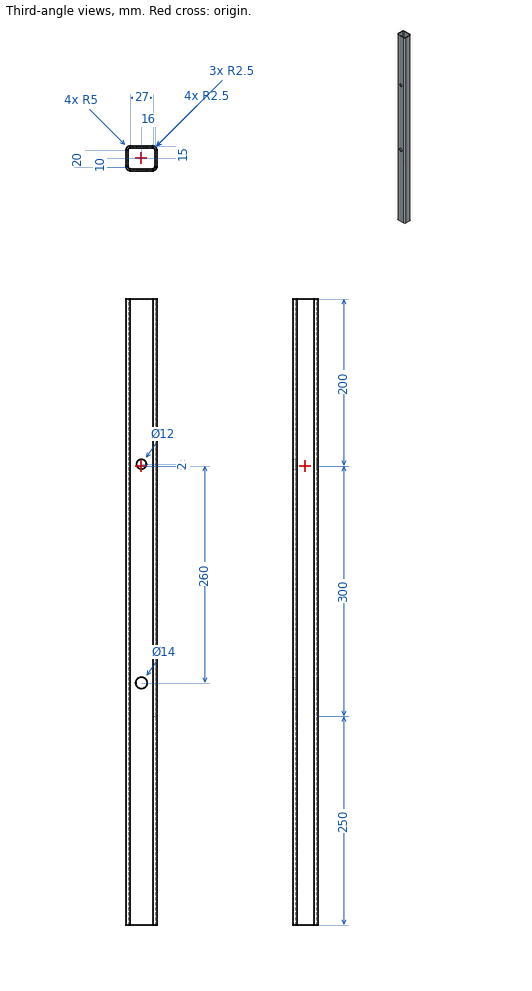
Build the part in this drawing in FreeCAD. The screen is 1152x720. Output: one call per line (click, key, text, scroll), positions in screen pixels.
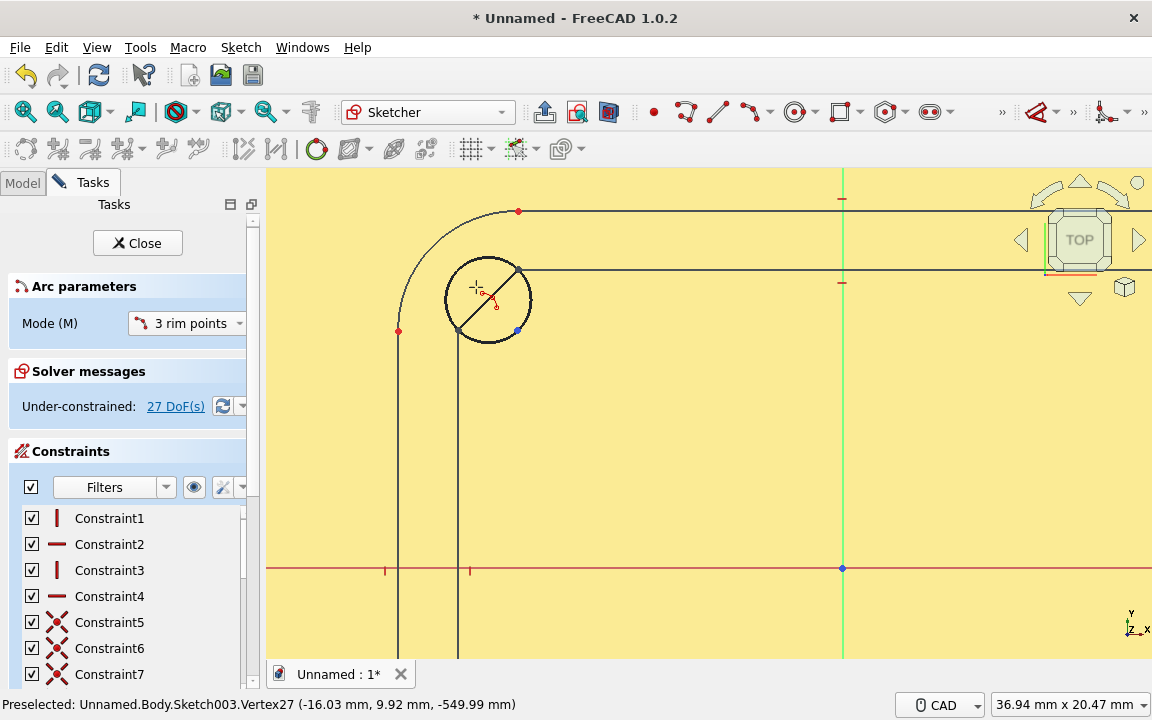
click(477, 286)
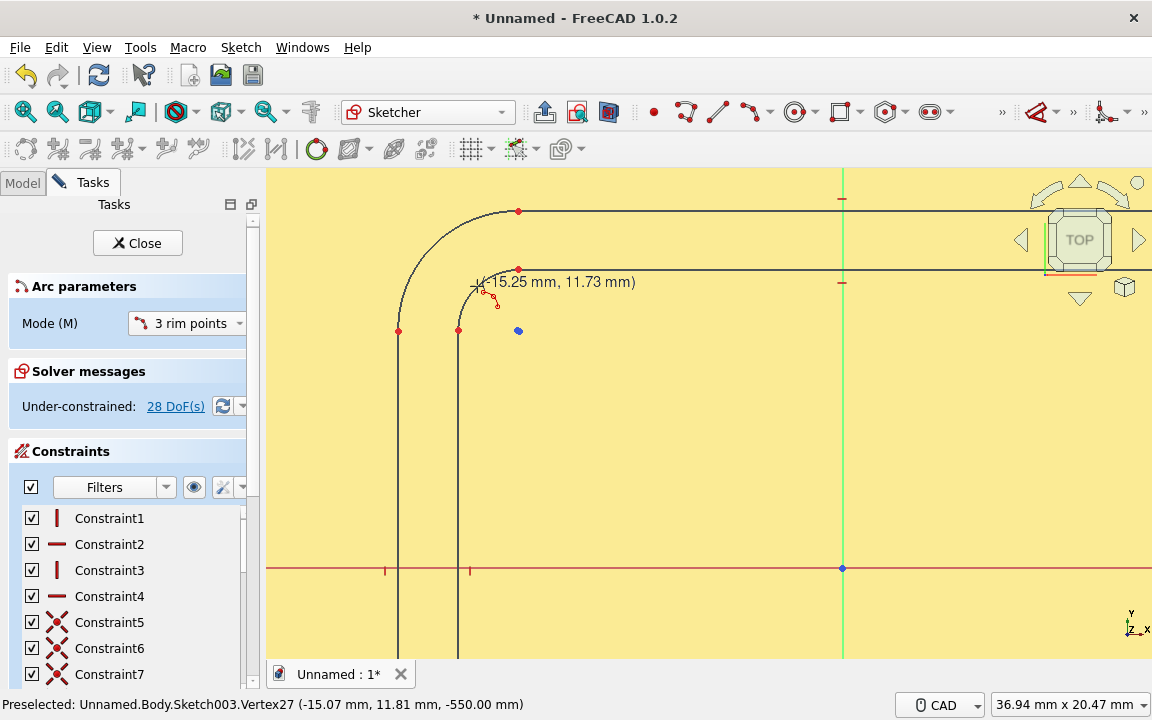
scroll(475, 287, down, 4)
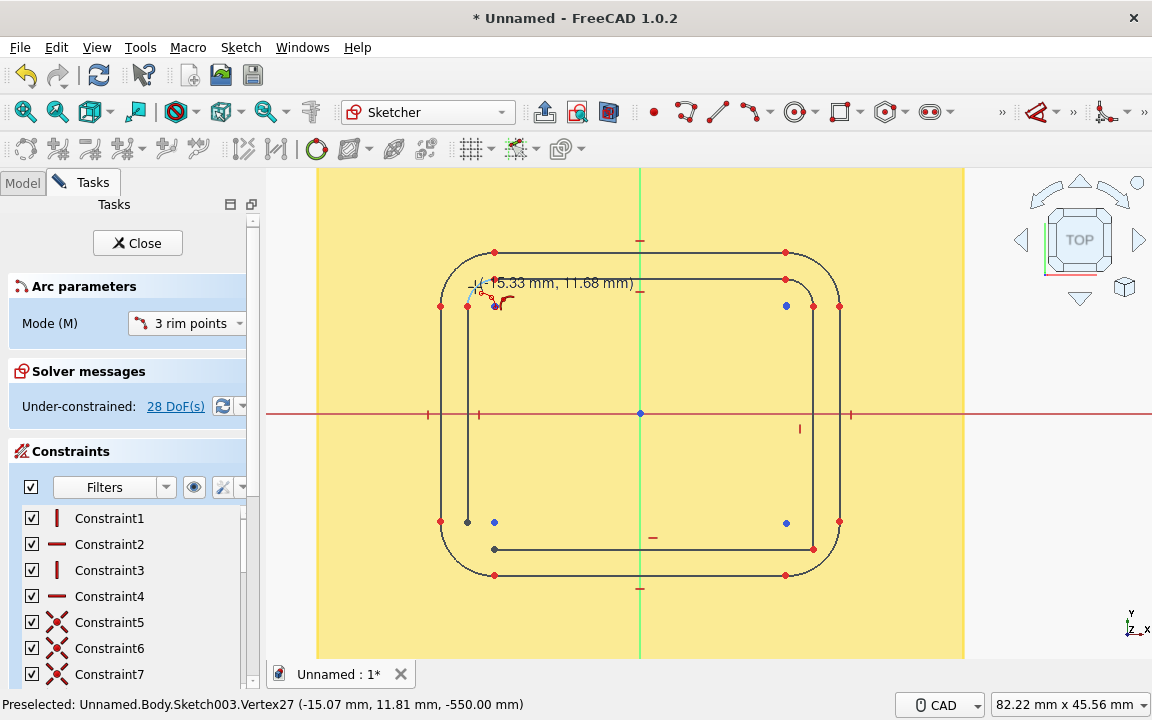
click(468, 522)
click(495, 550)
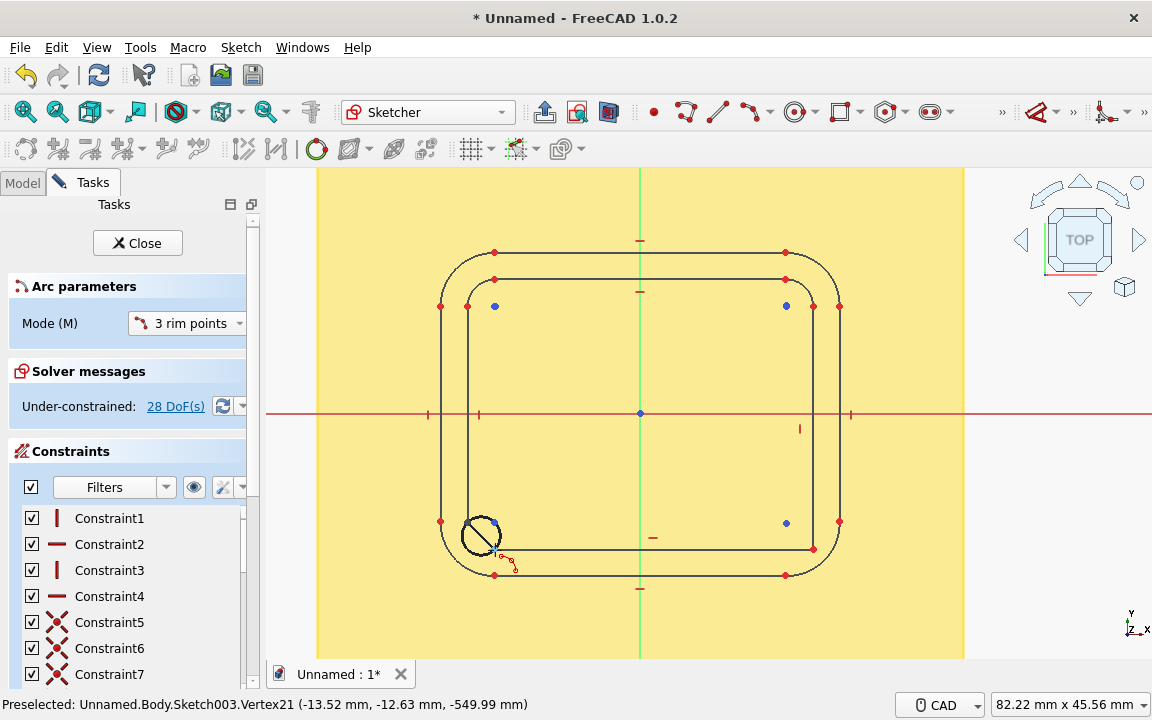
scroll(476, 540, up, 4)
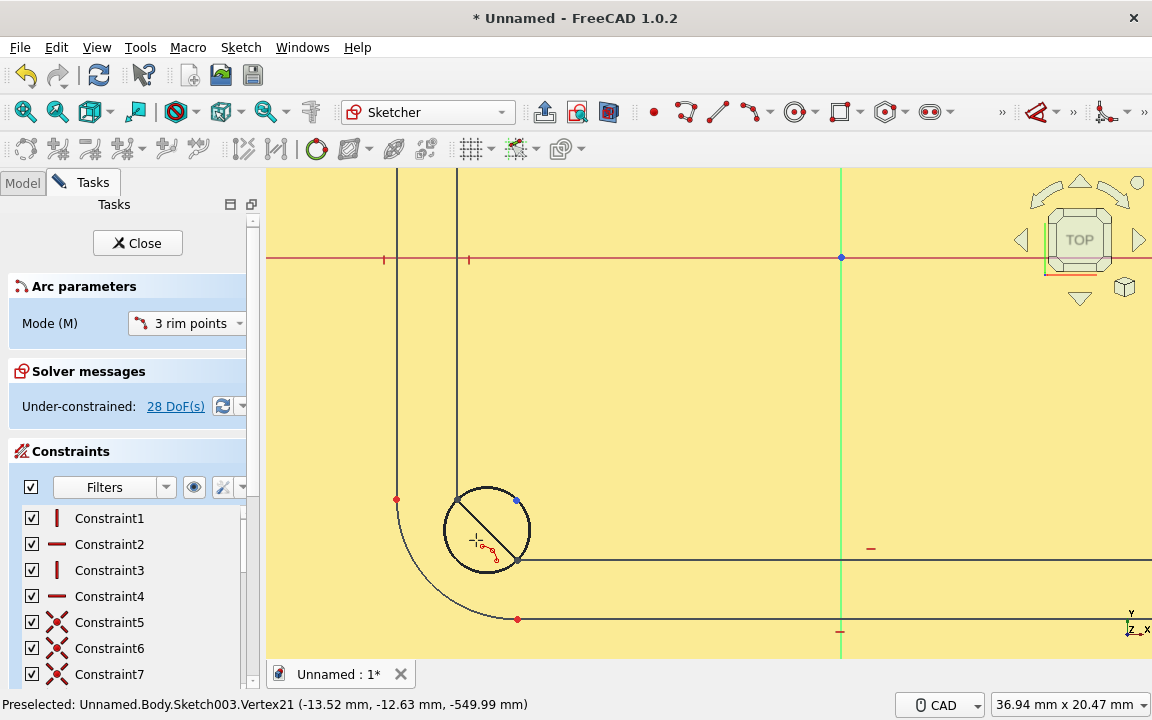
click(475, 540)
key(Escape)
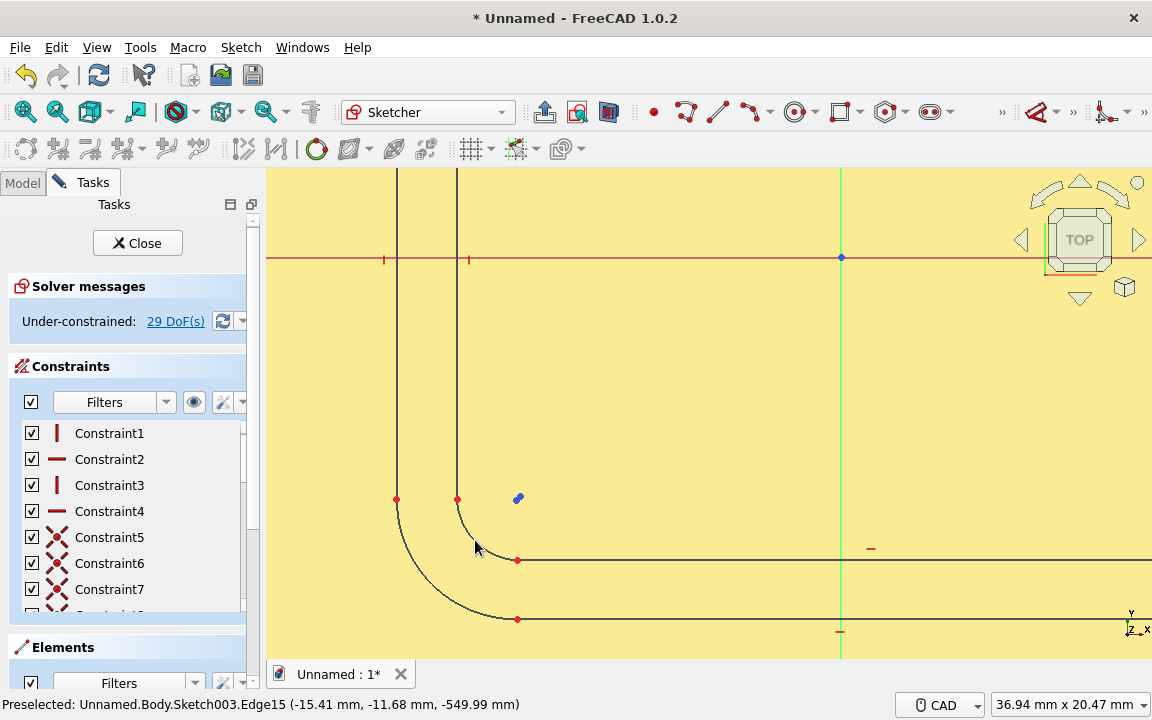
click(397, 355)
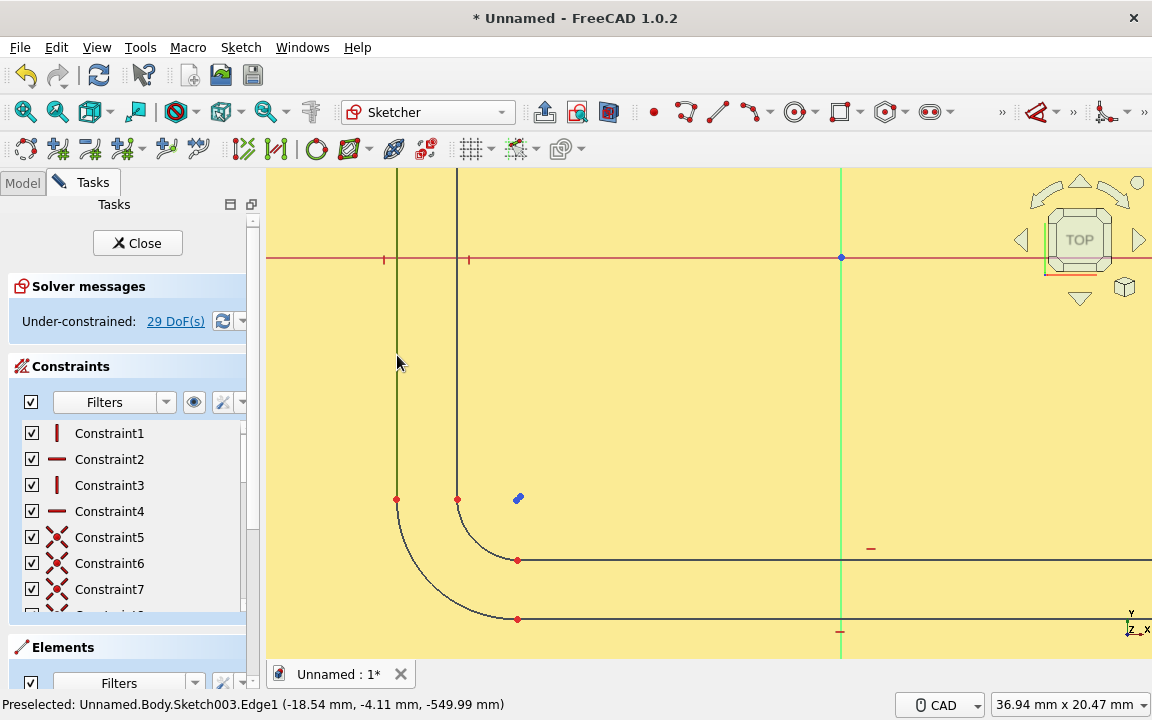
scroll(476, 541, down, 4)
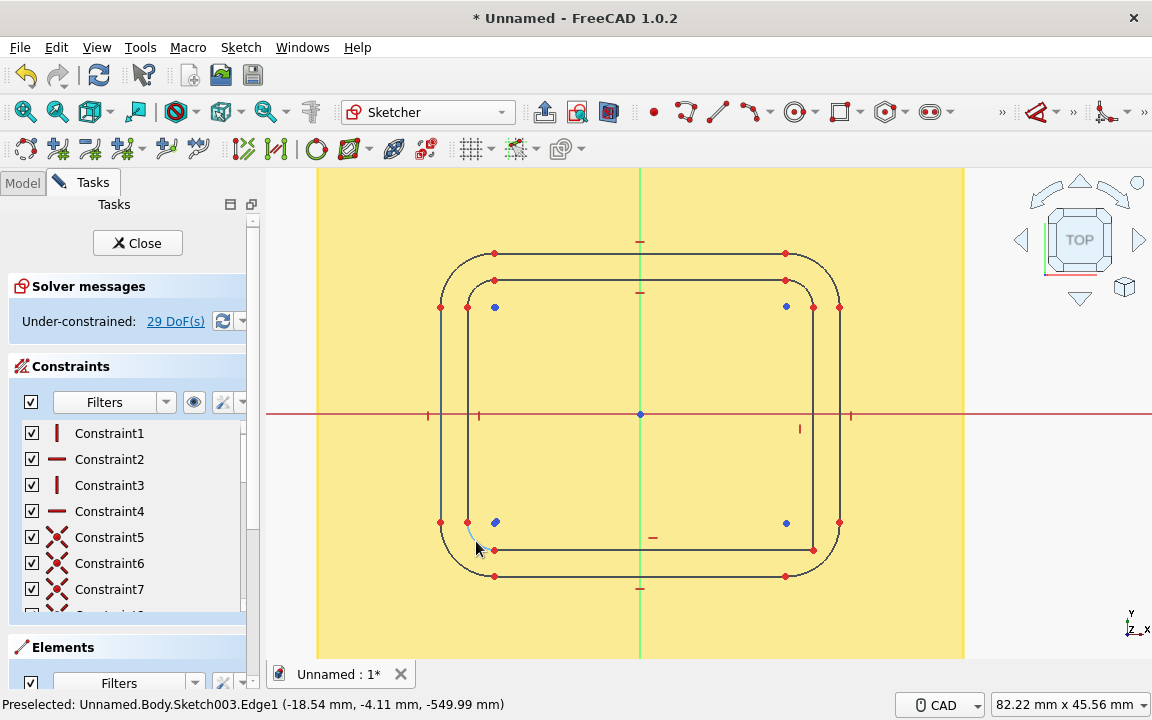
click(470, 259)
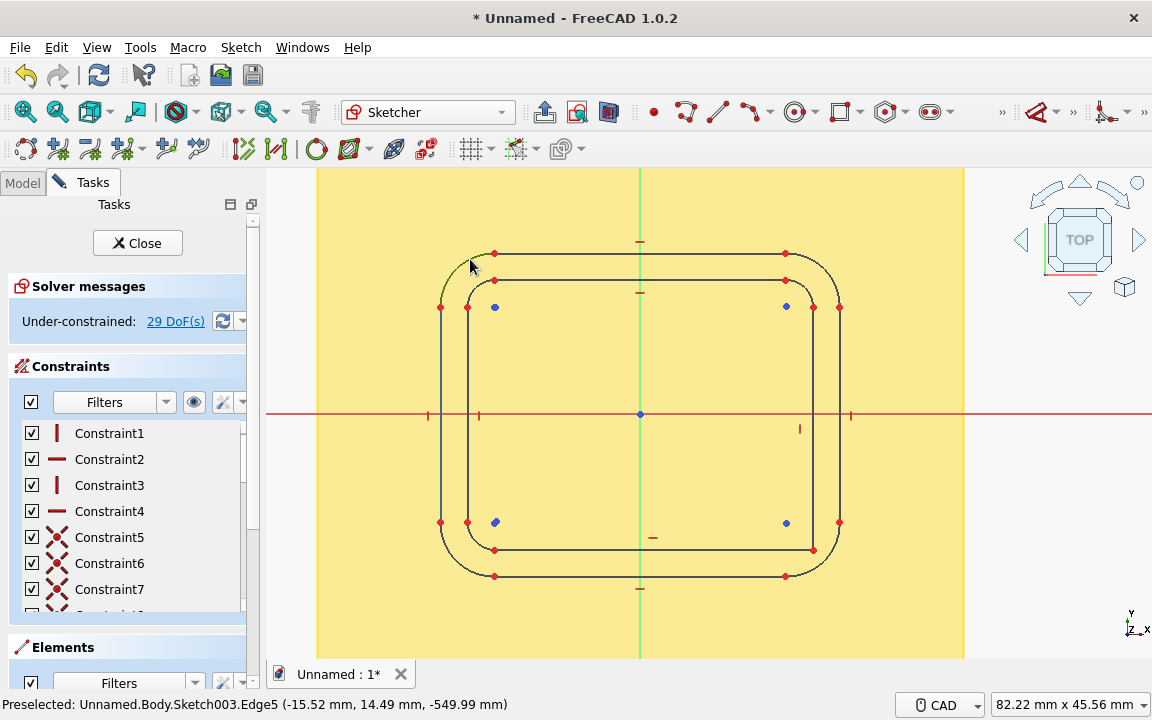
key(t)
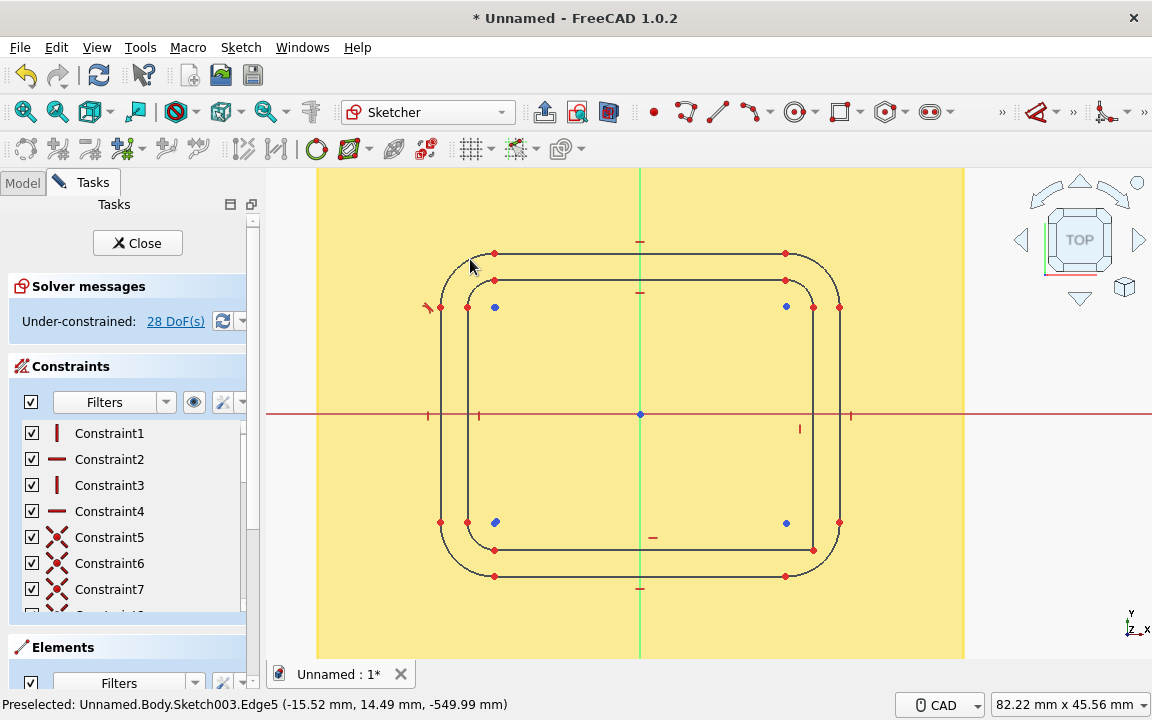
click(441, 458)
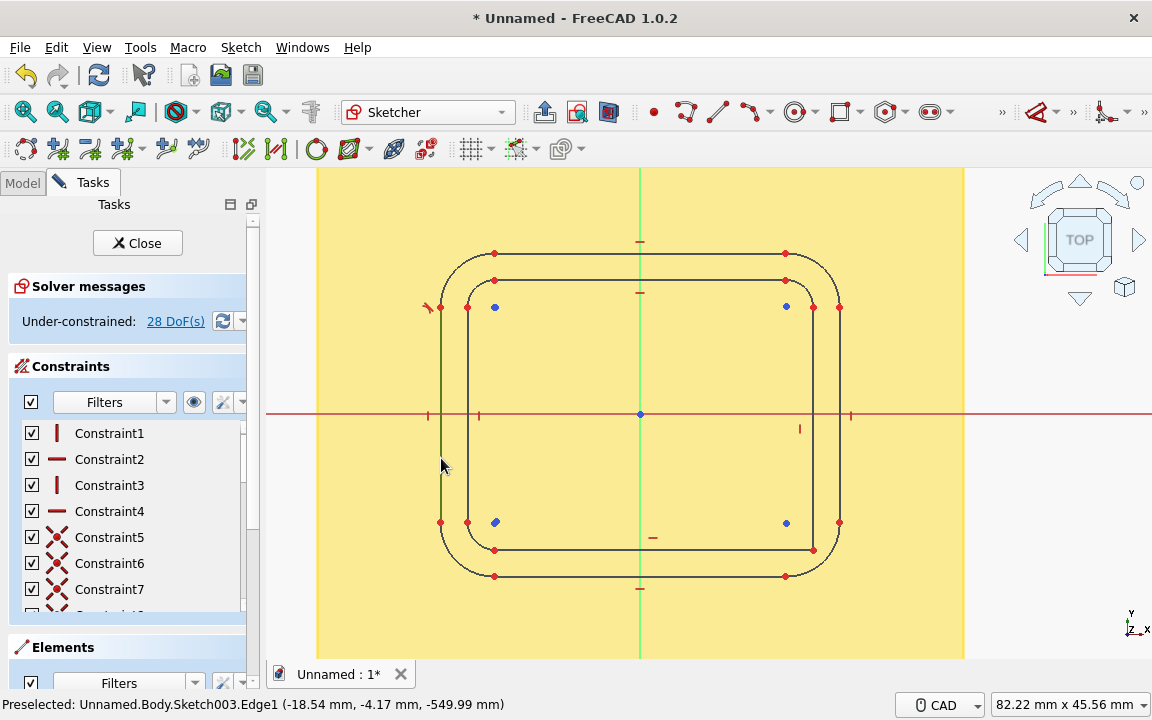
click(446, 547)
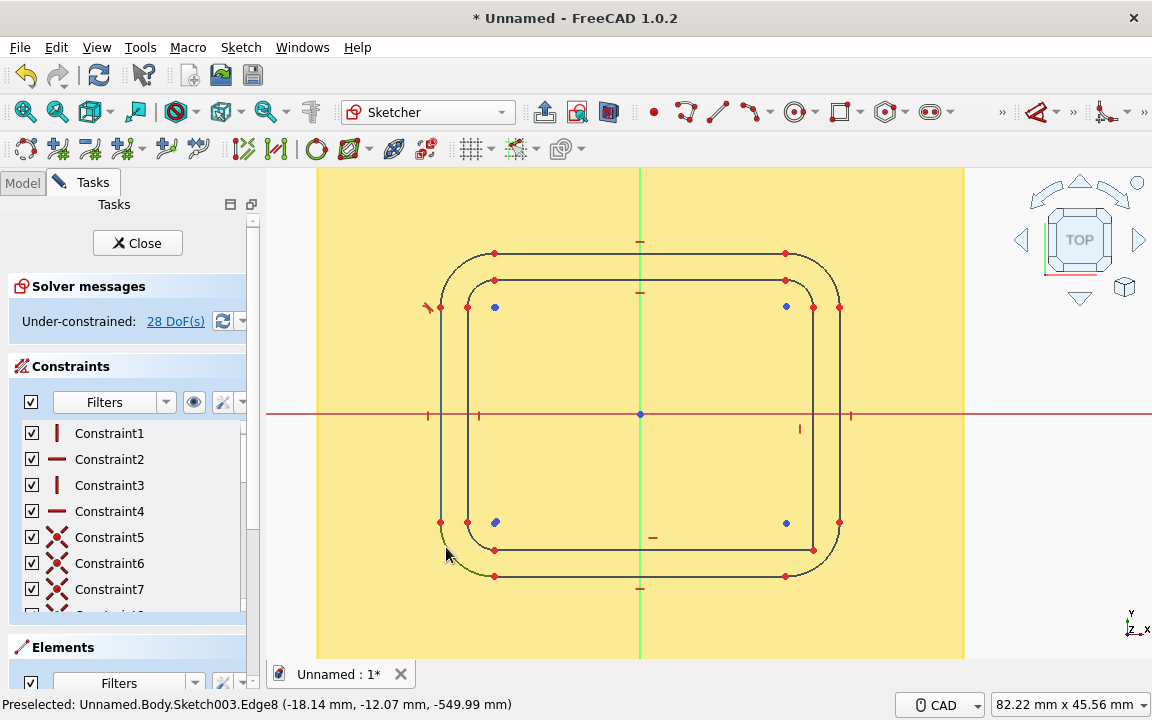
key(t)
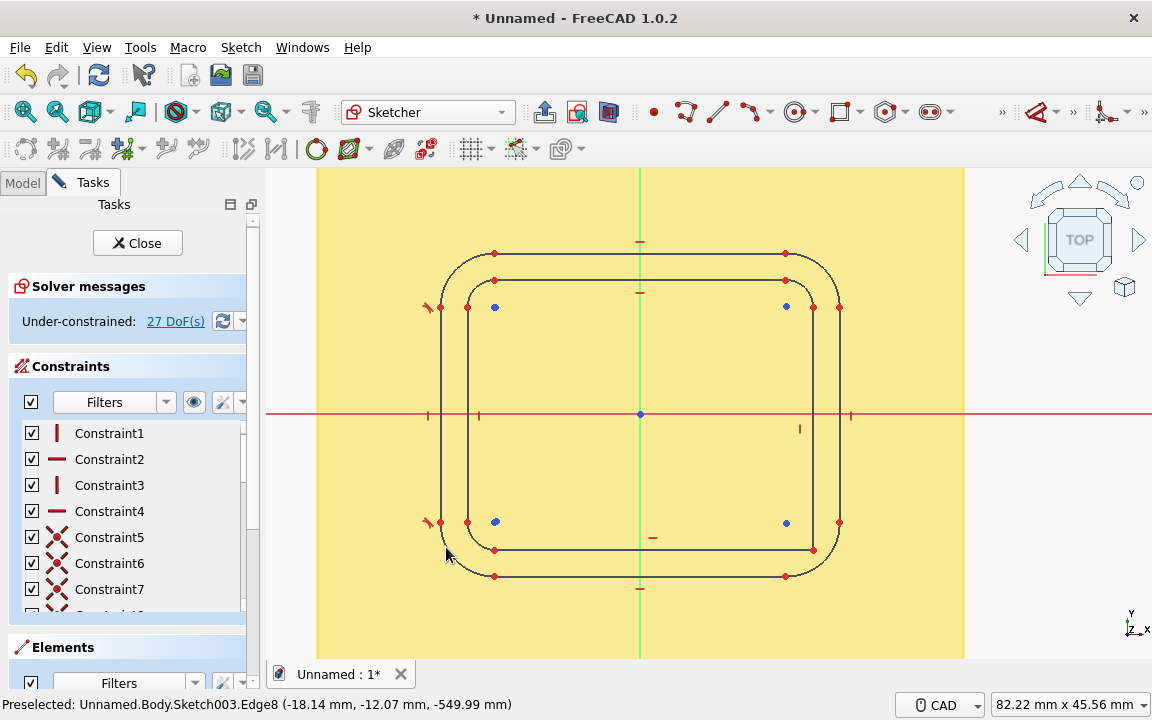
click(582, 254)